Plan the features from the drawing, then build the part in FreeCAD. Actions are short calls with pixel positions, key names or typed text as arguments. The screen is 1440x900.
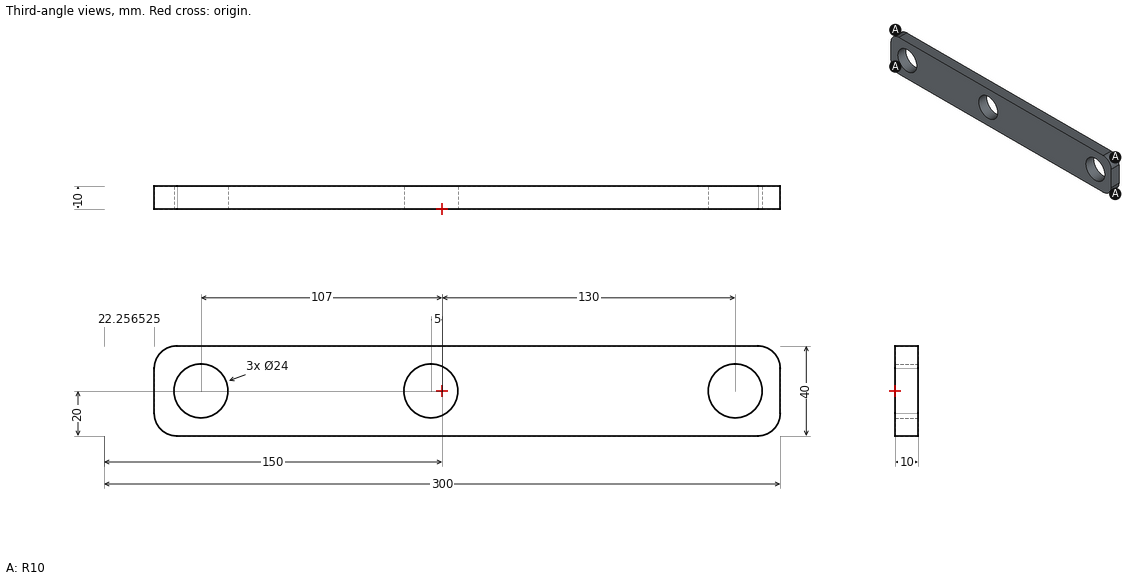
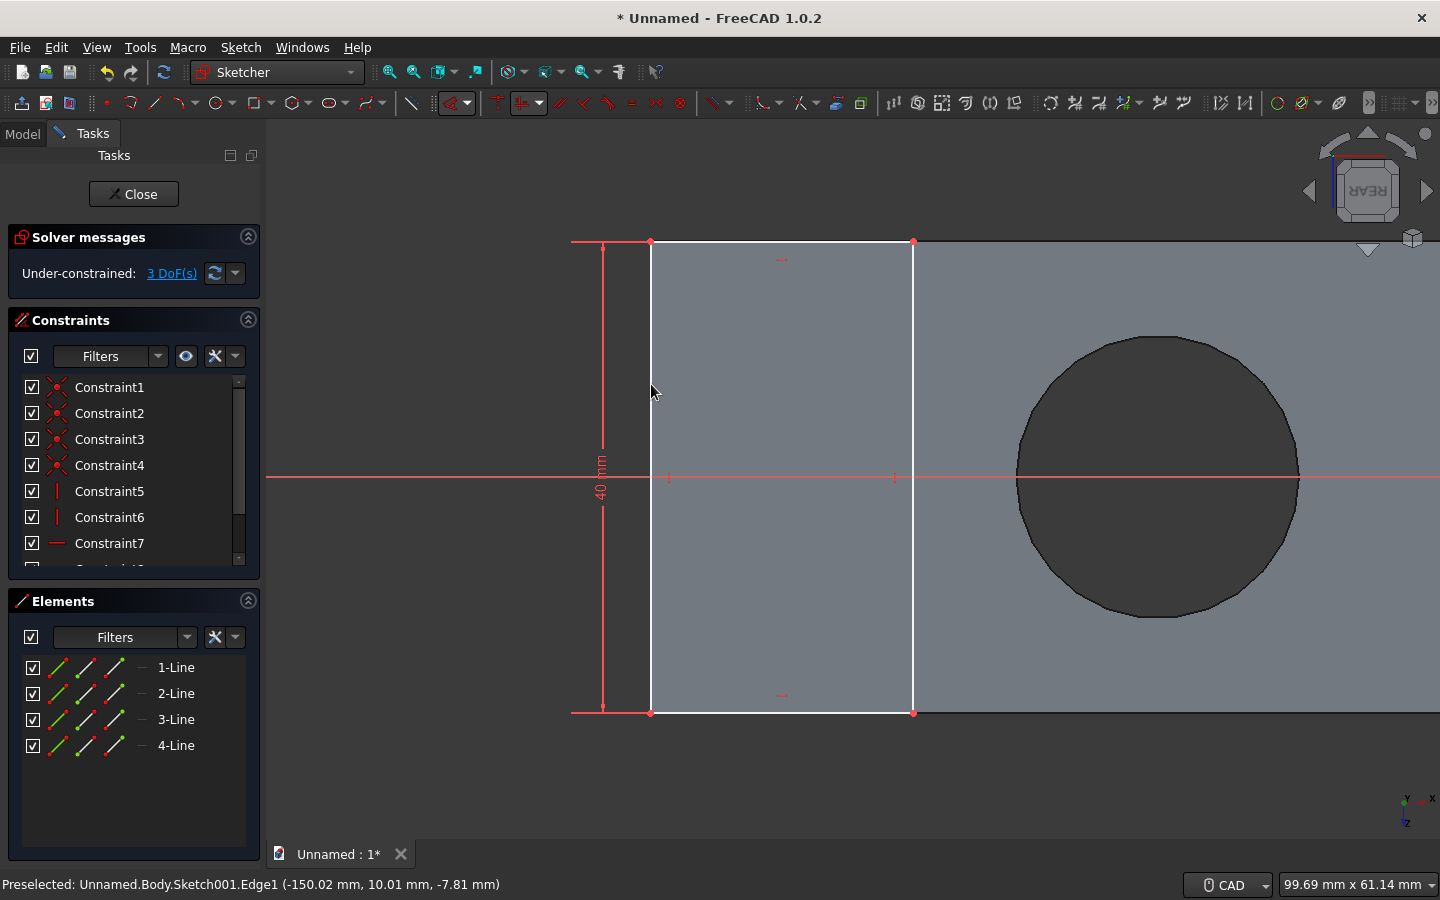
click(651, 242)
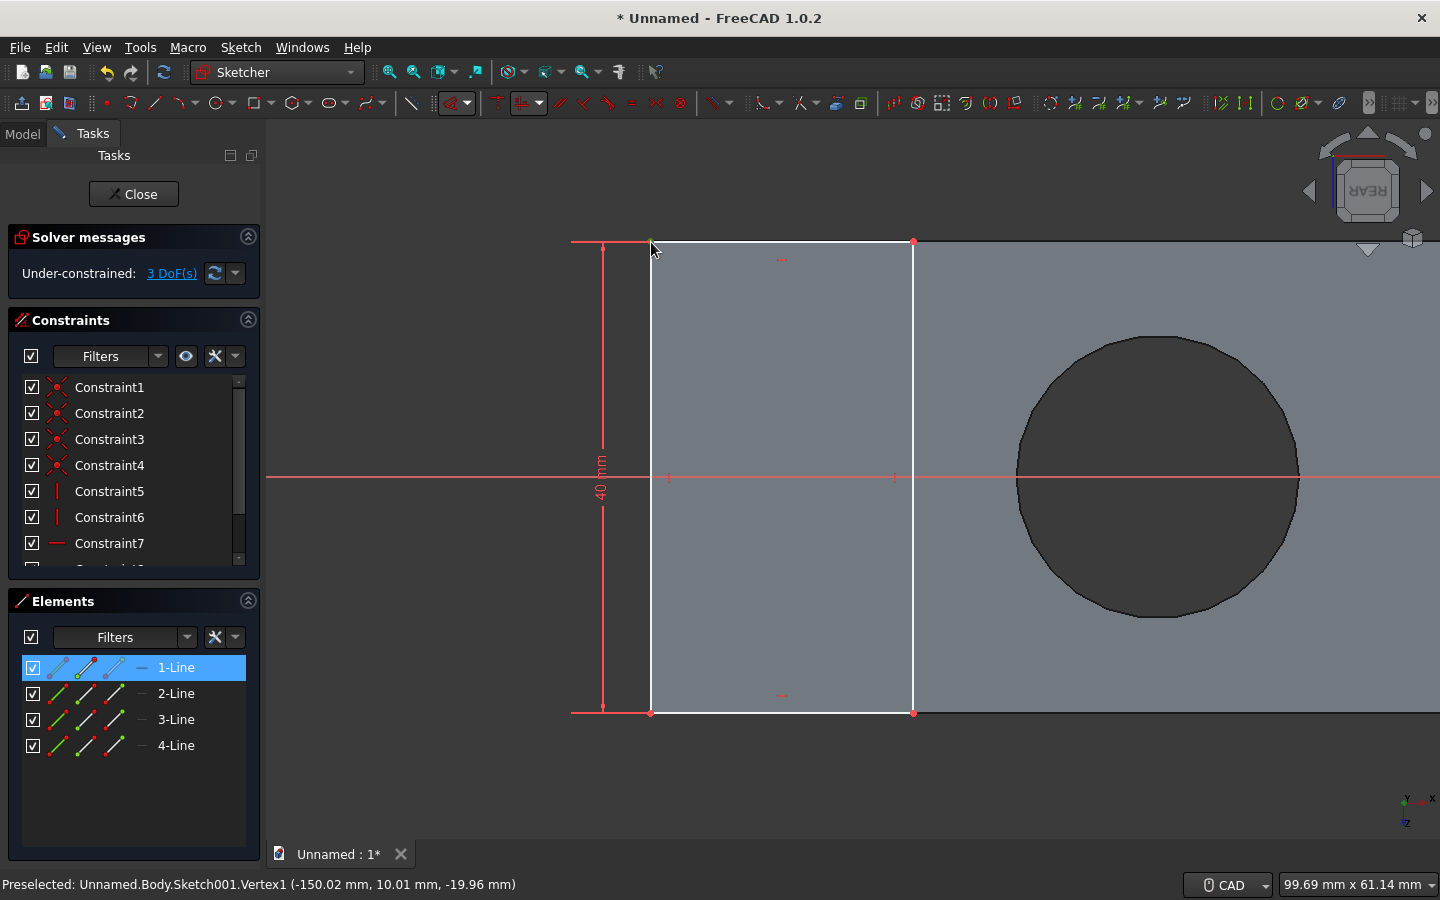
key(i)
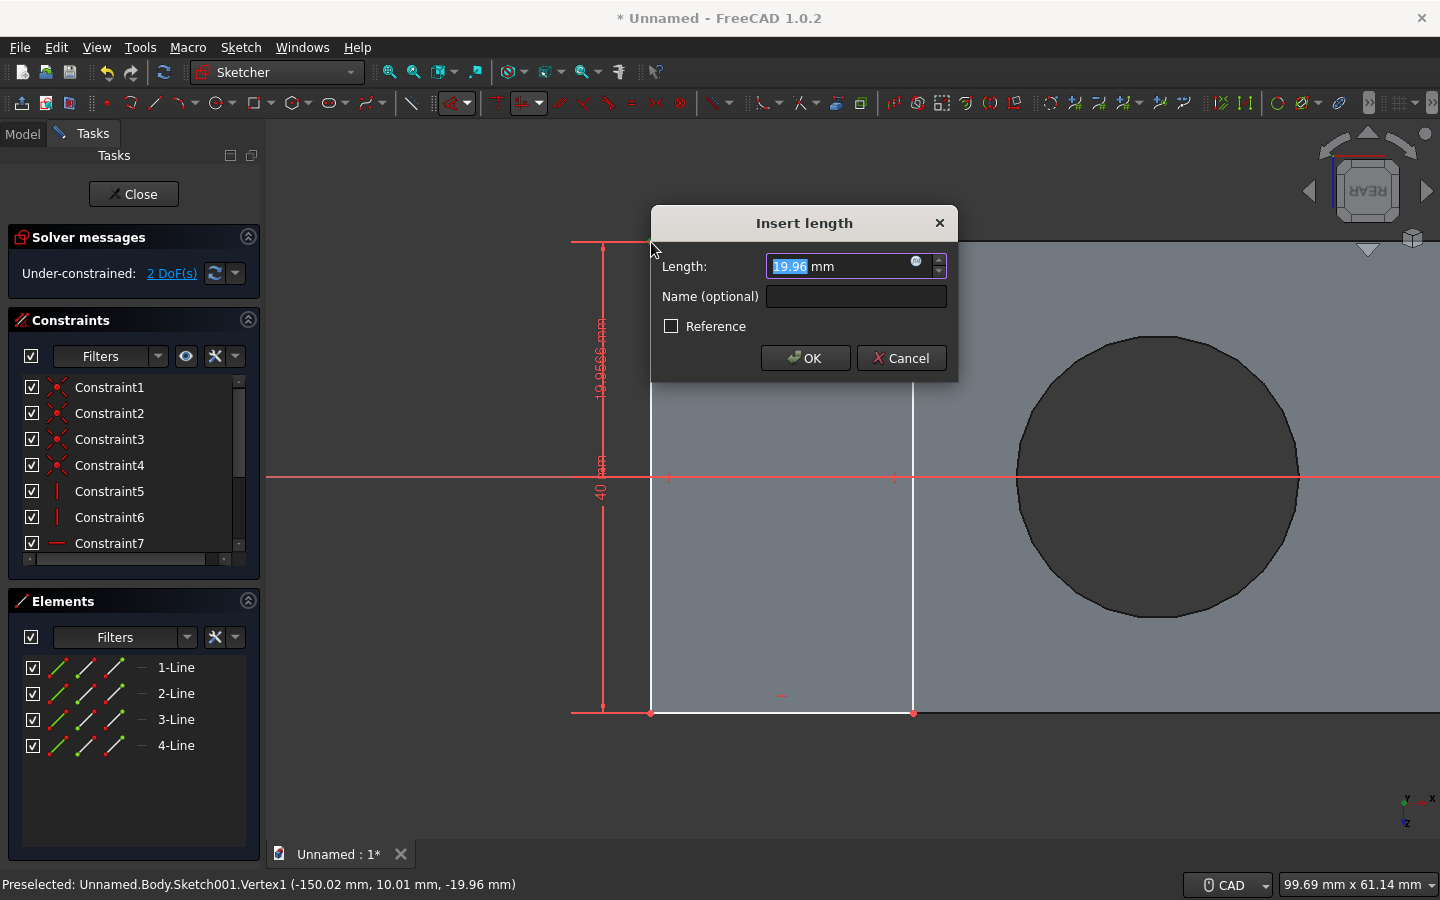
text(20)
key(Return)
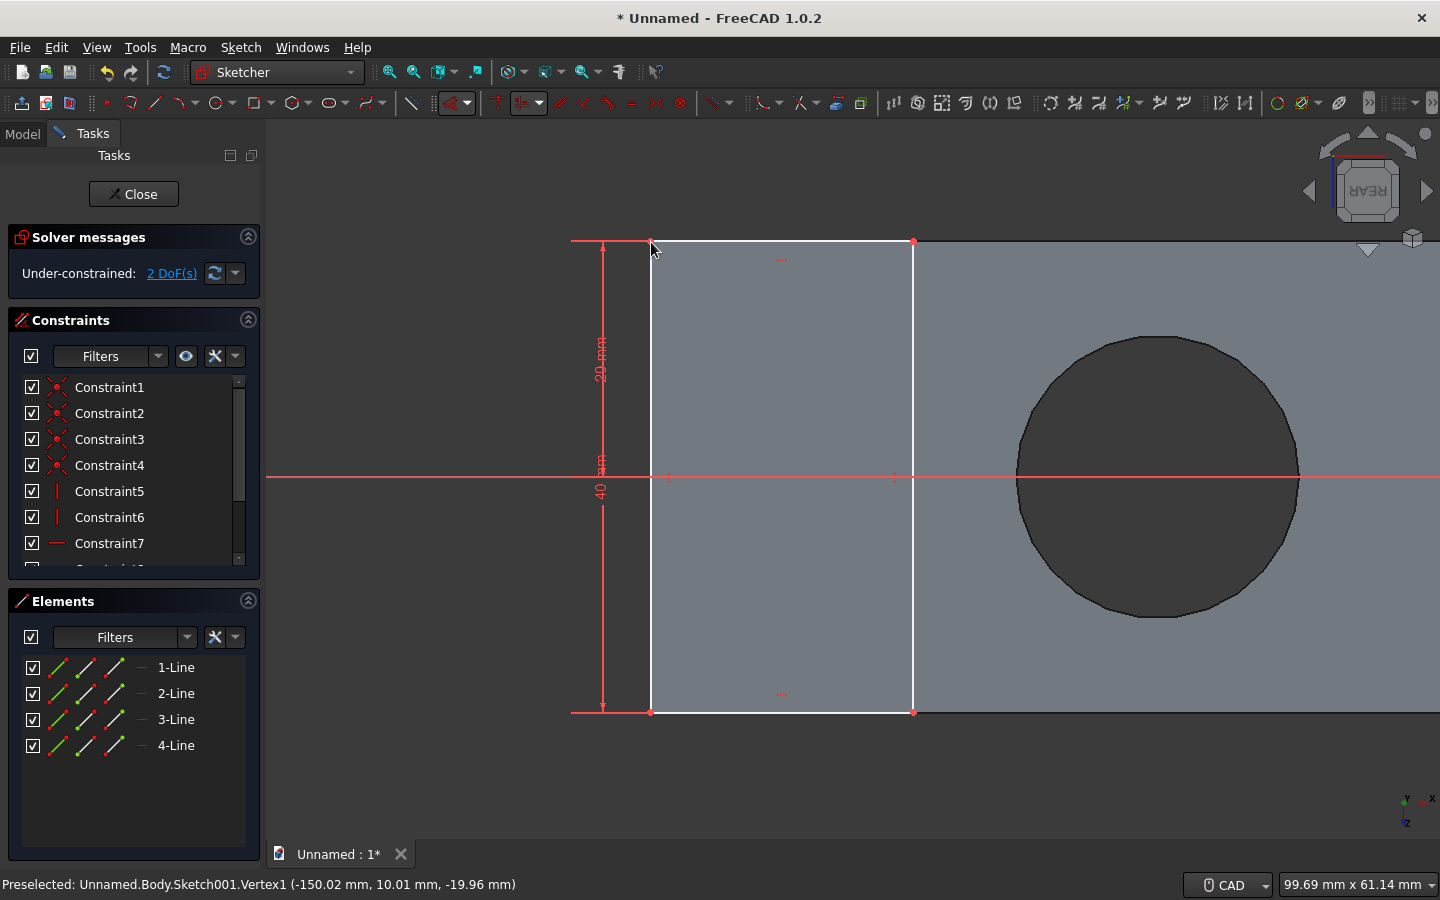
click(651, 241)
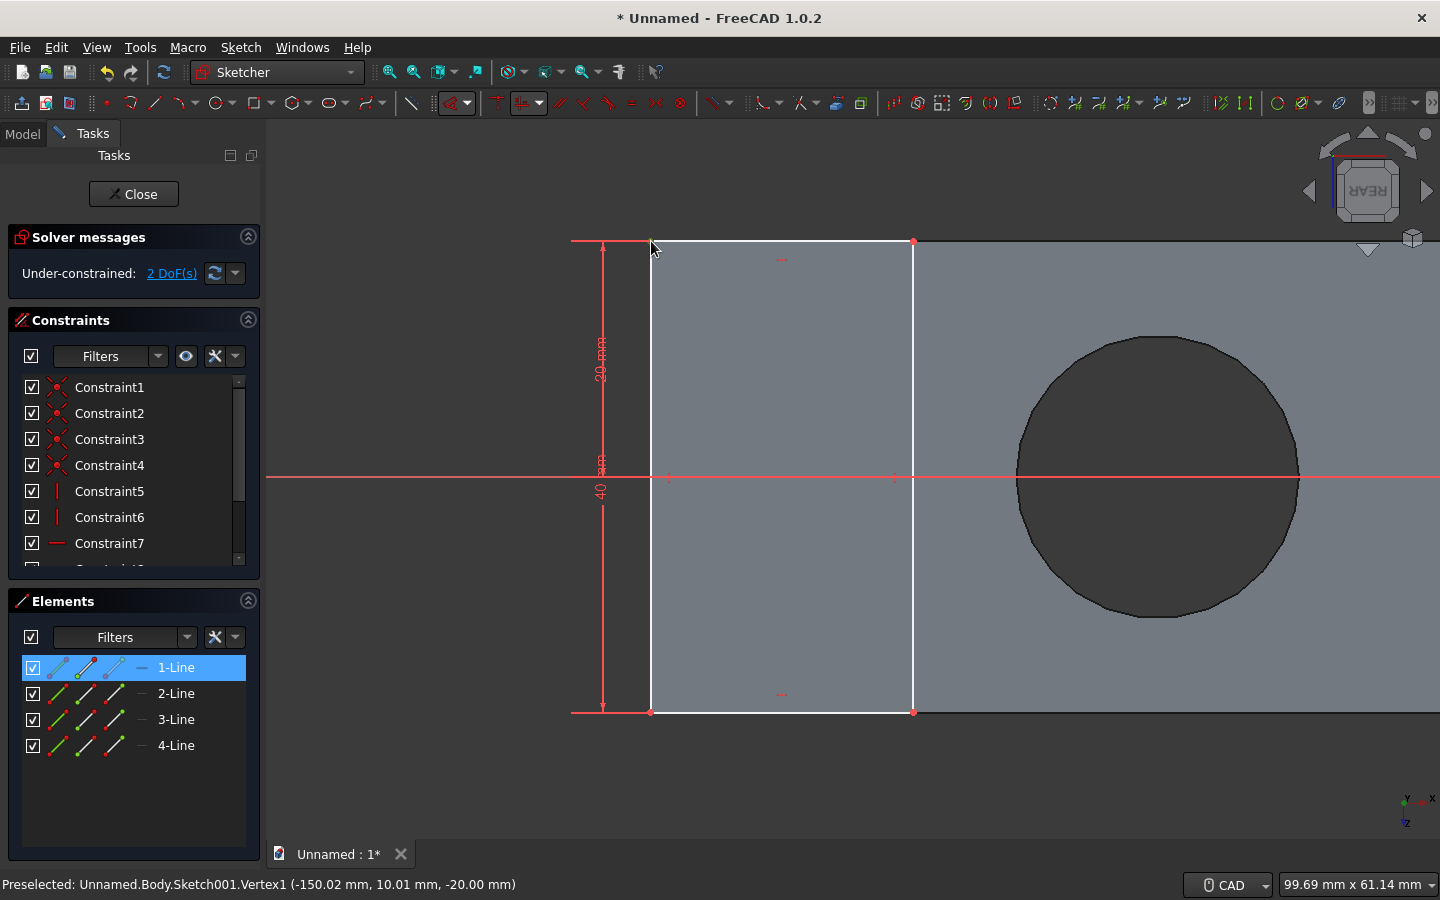
click(470, 104)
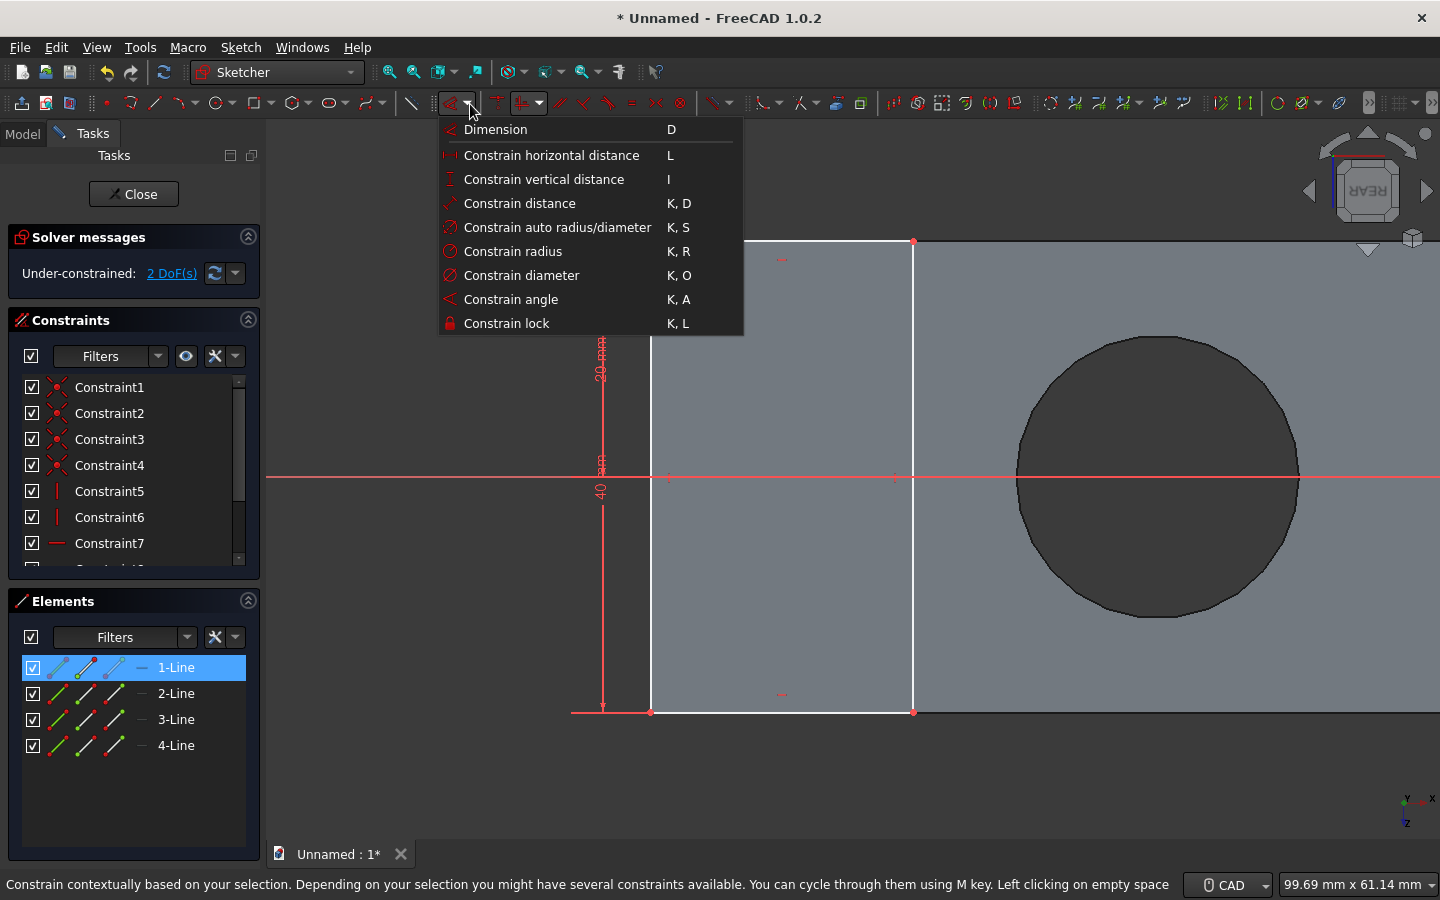
click(591, 155)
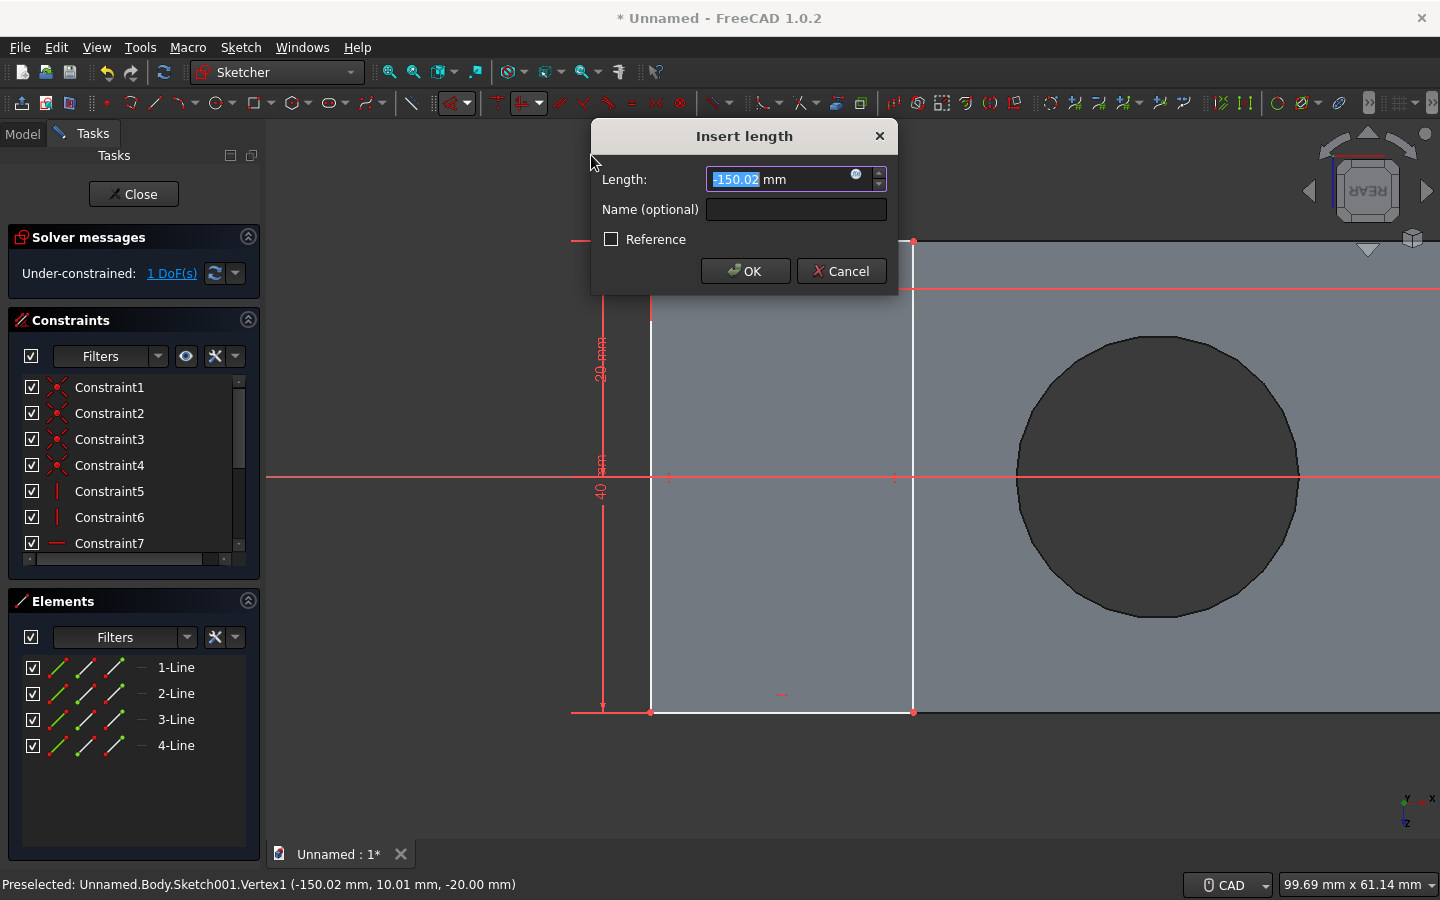
text(-150)
key(Return)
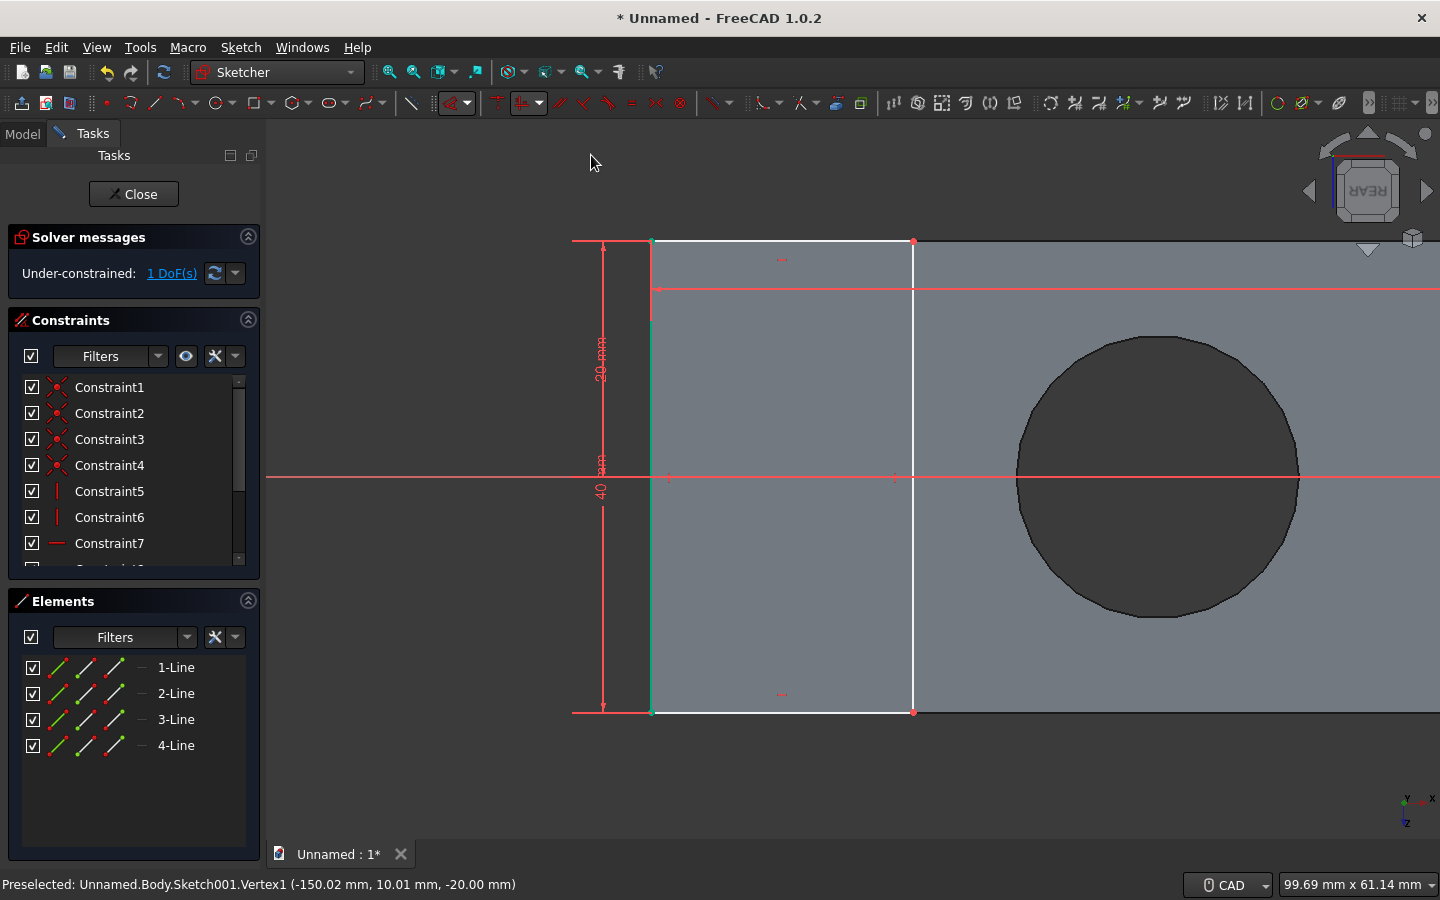
click(730, 713)